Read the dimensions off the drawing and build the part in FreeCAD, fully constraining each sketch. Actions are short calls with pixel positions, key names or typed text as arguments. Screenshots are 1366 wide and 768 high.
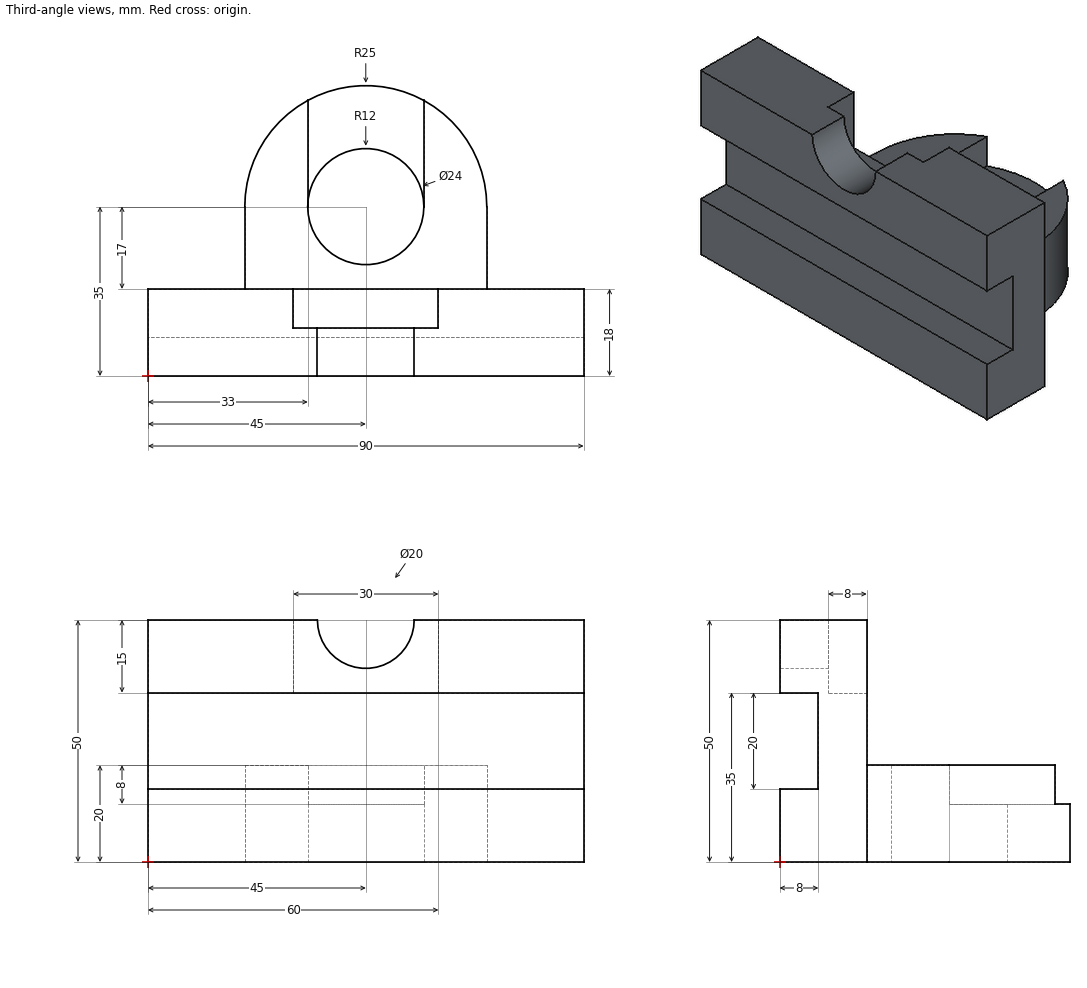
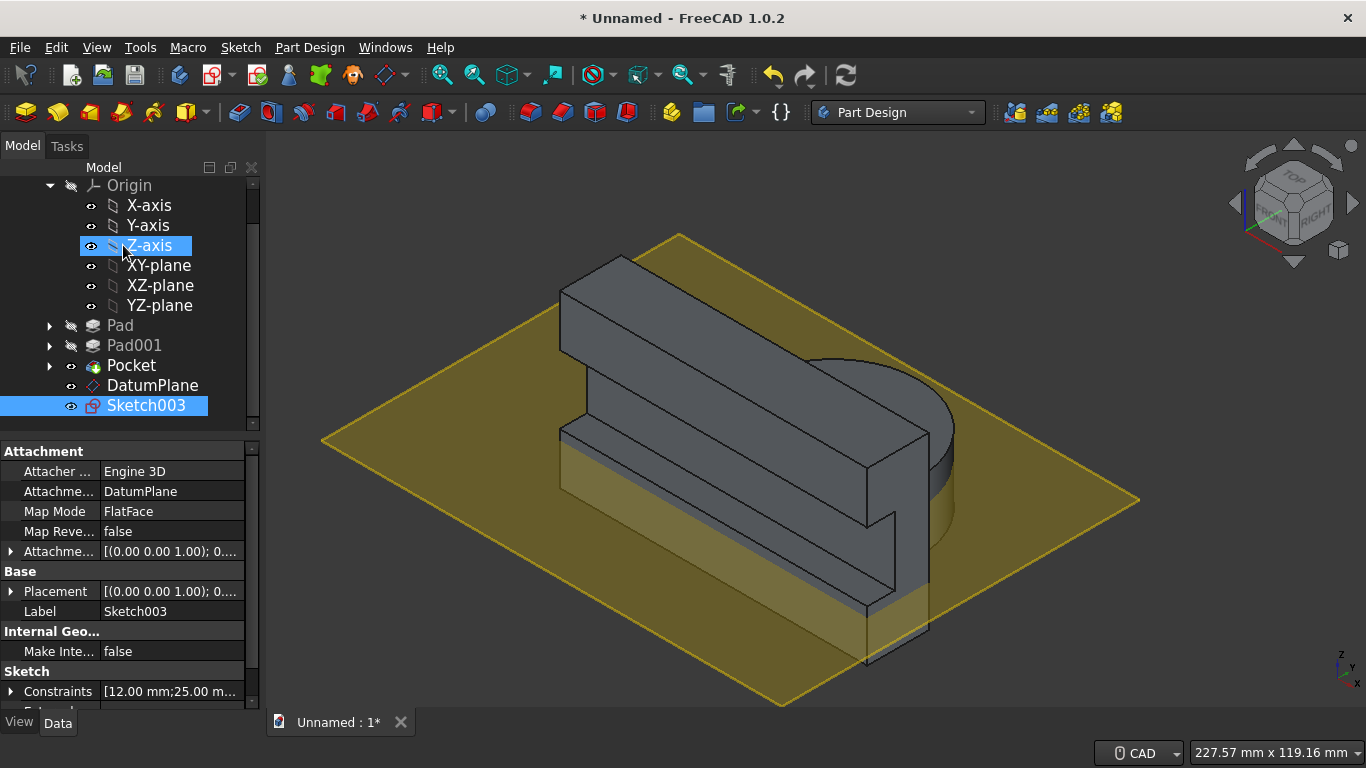
click(240, 112)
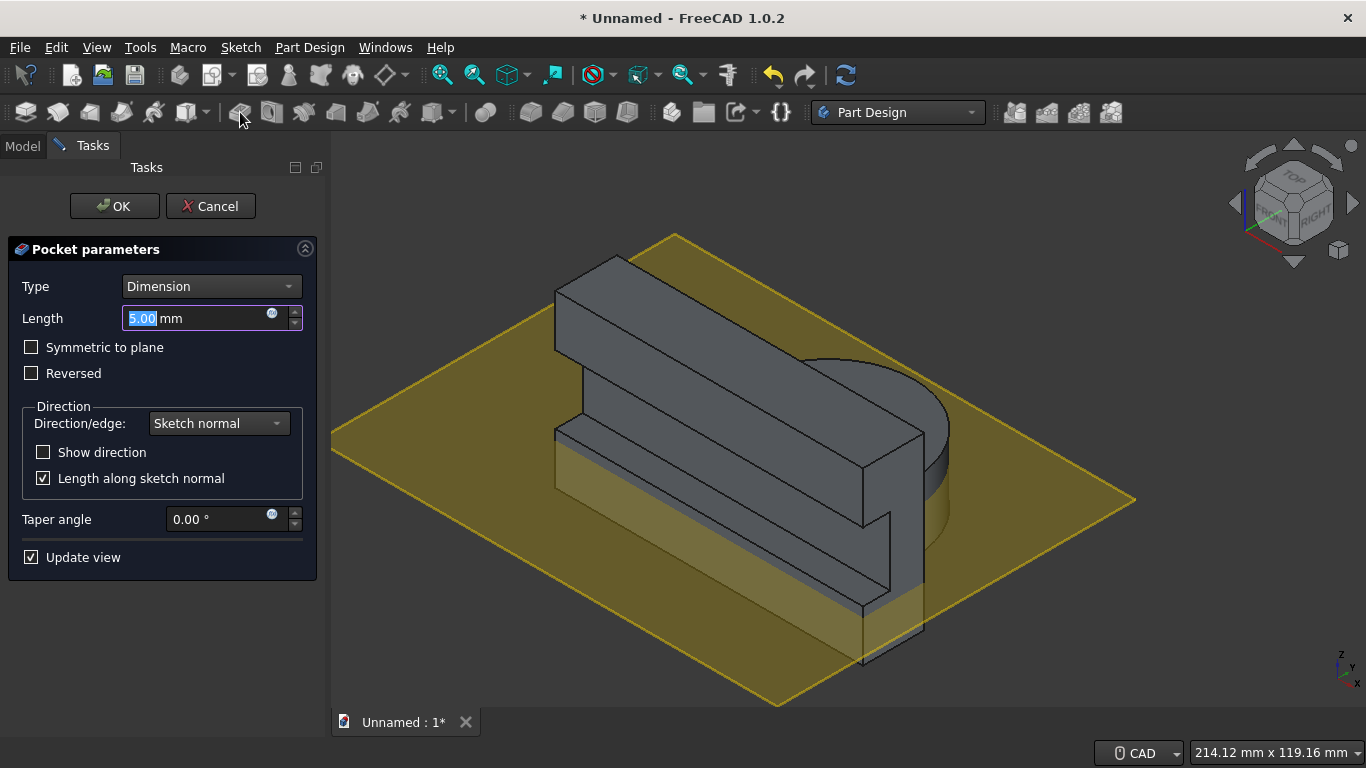
text(8)
key(Tab)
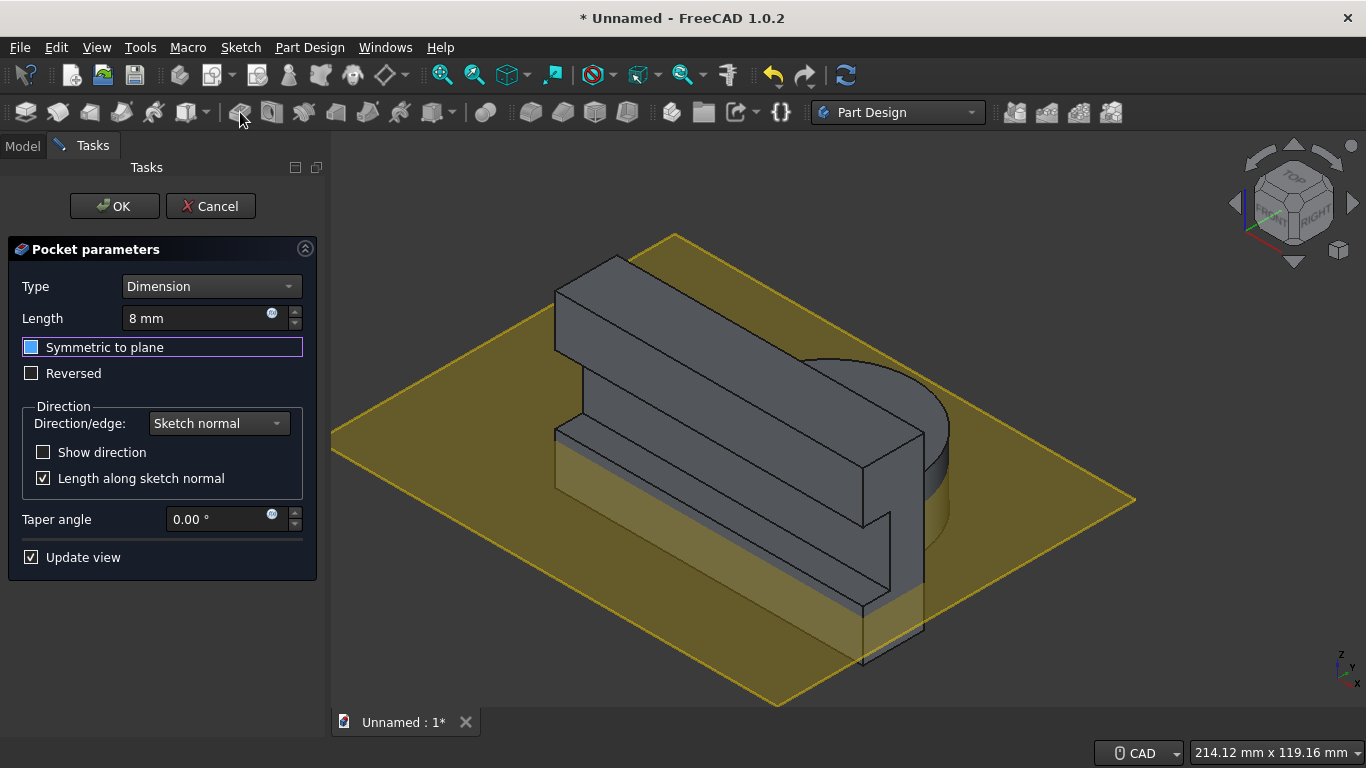
click(30, 373)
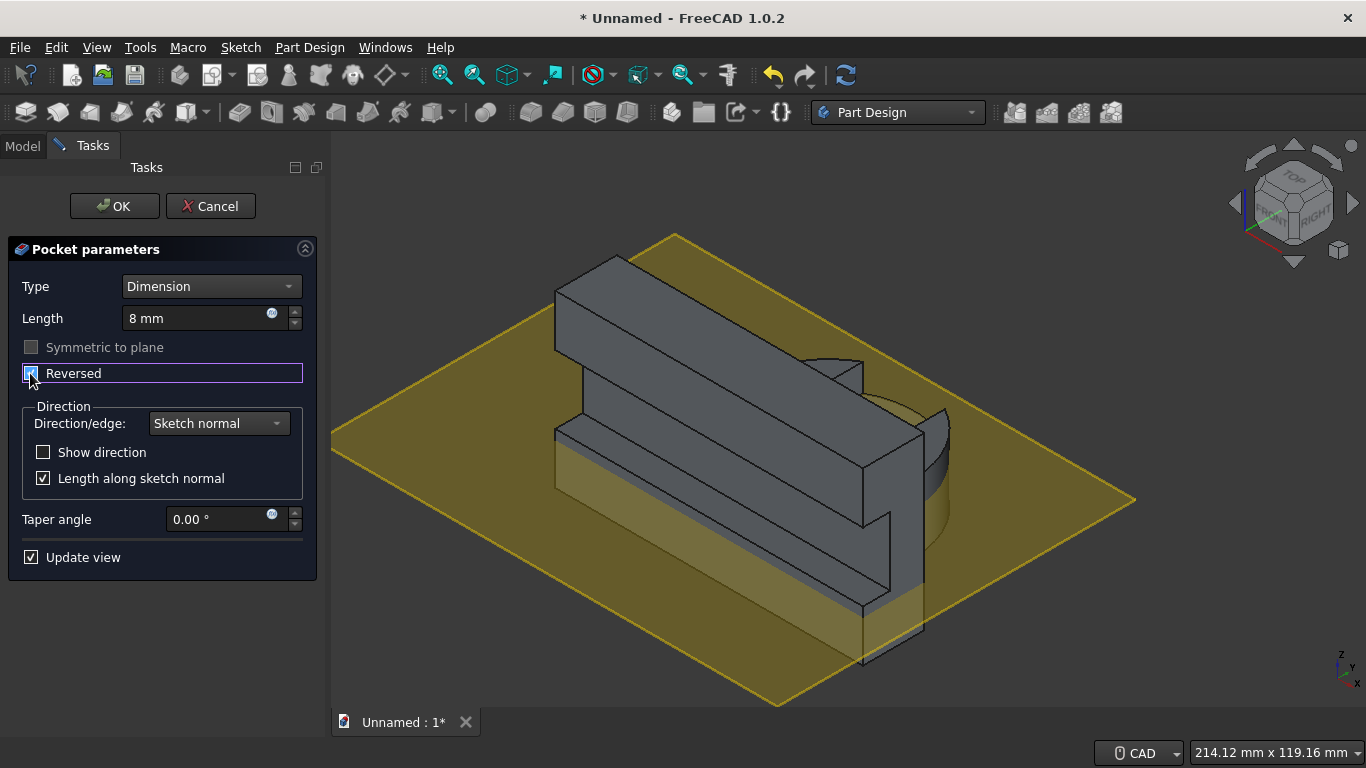
click(115, 206)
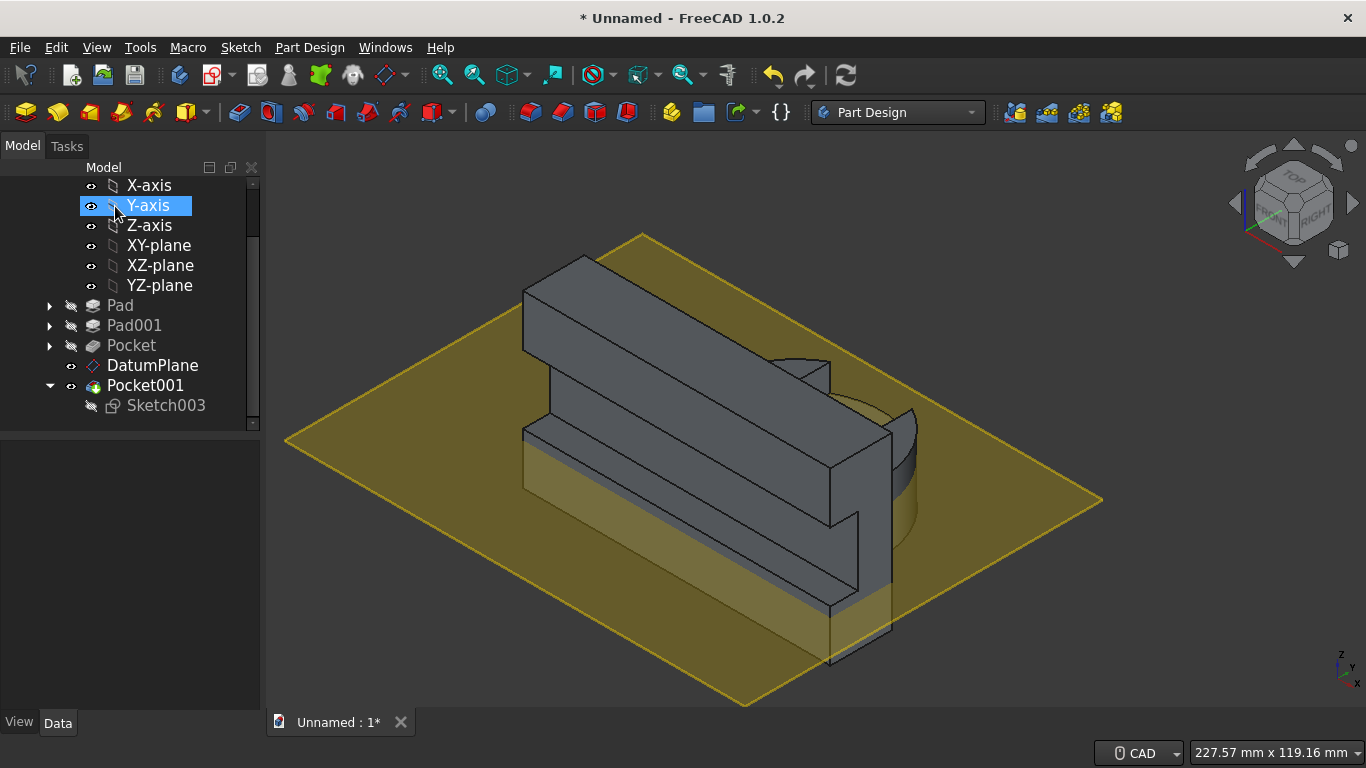
click(116, 366)
key(space)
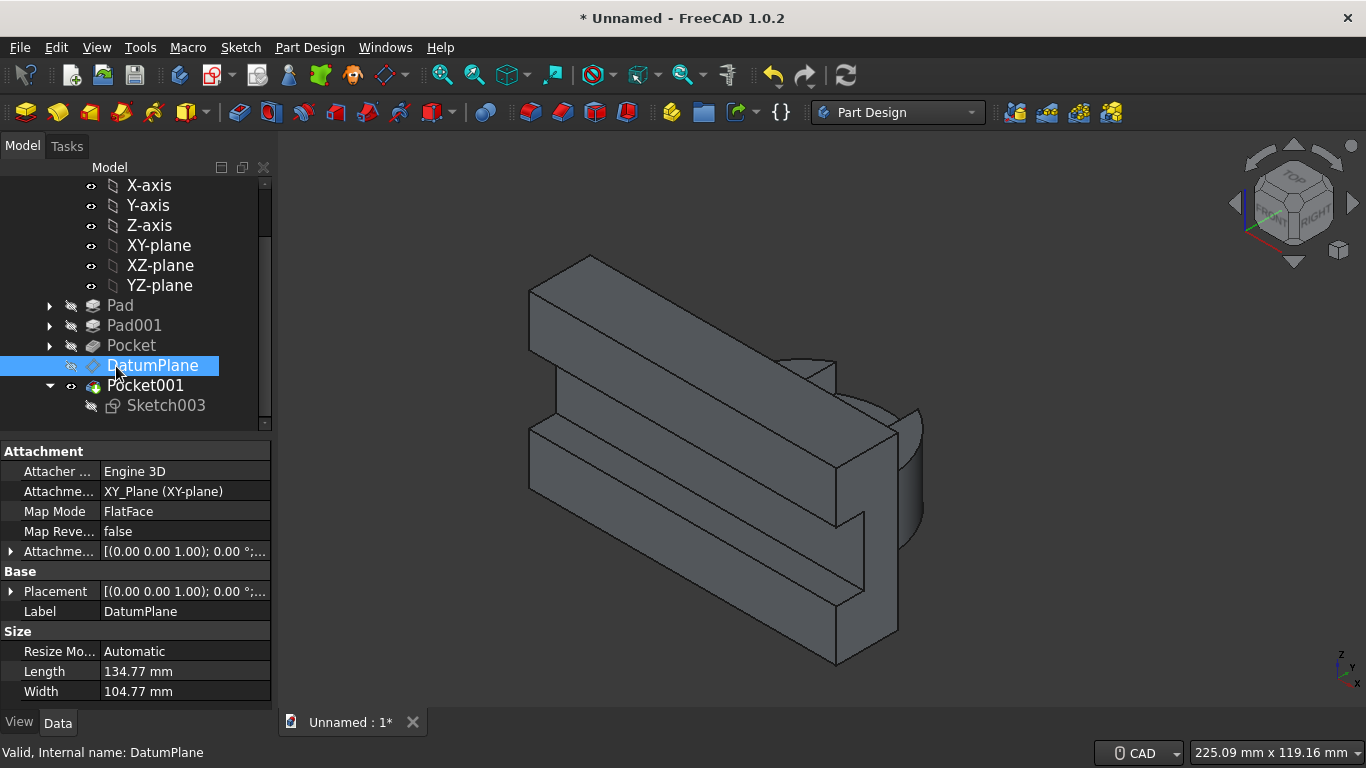
key(4)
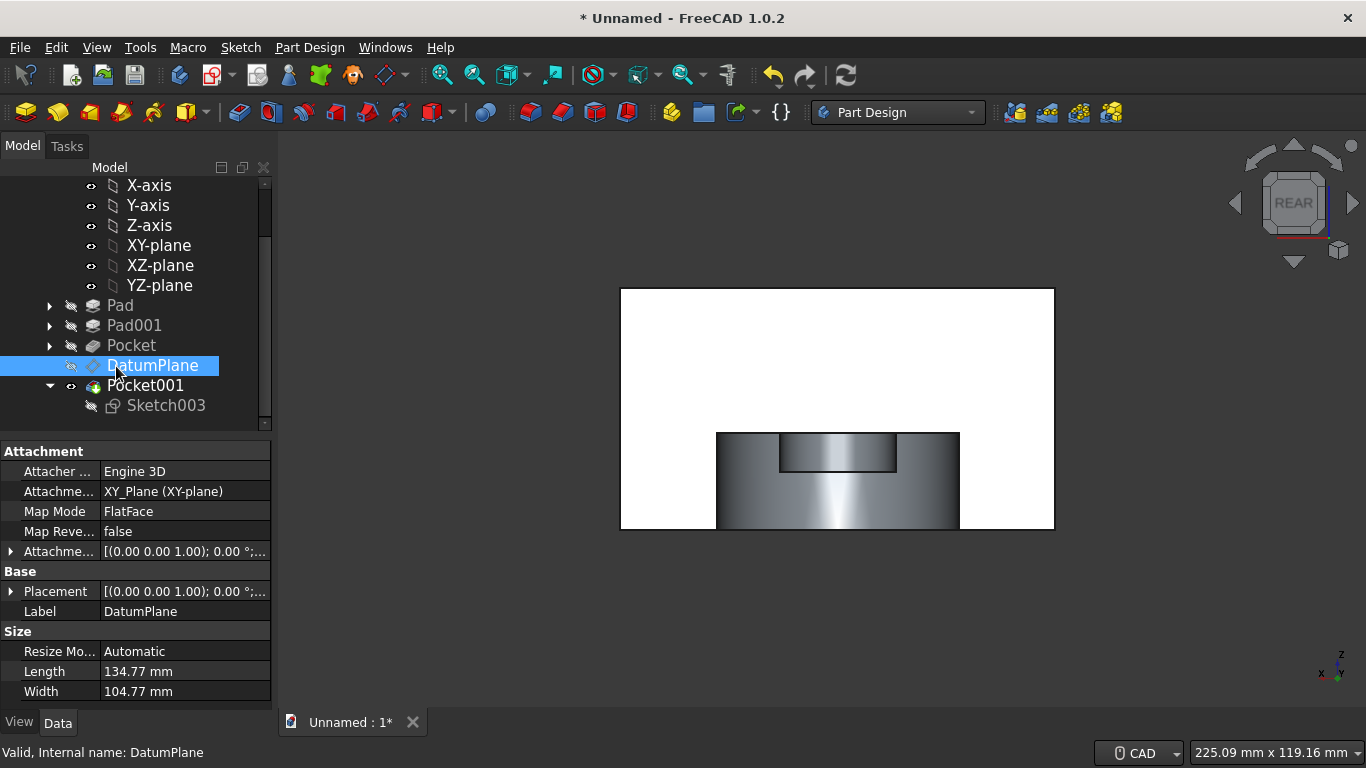
click(444, 76)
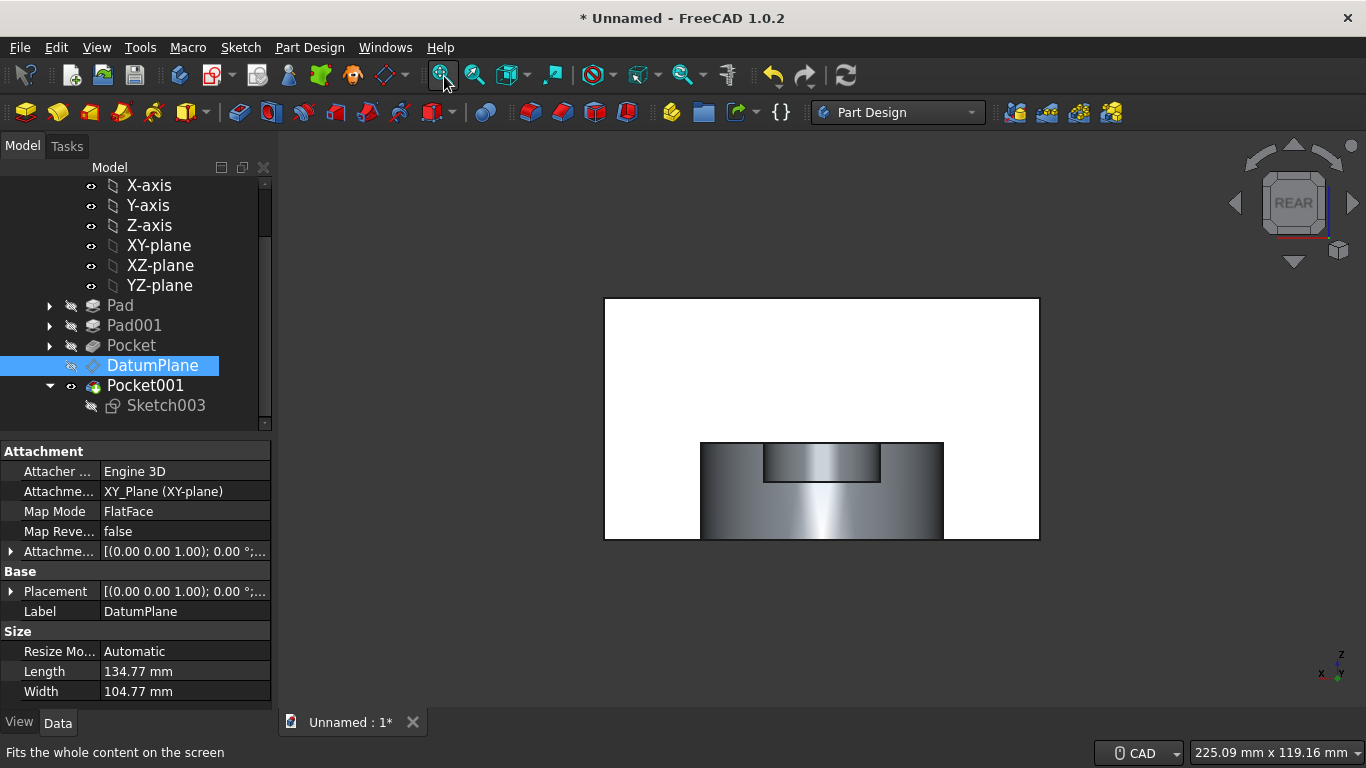
click(698, 383)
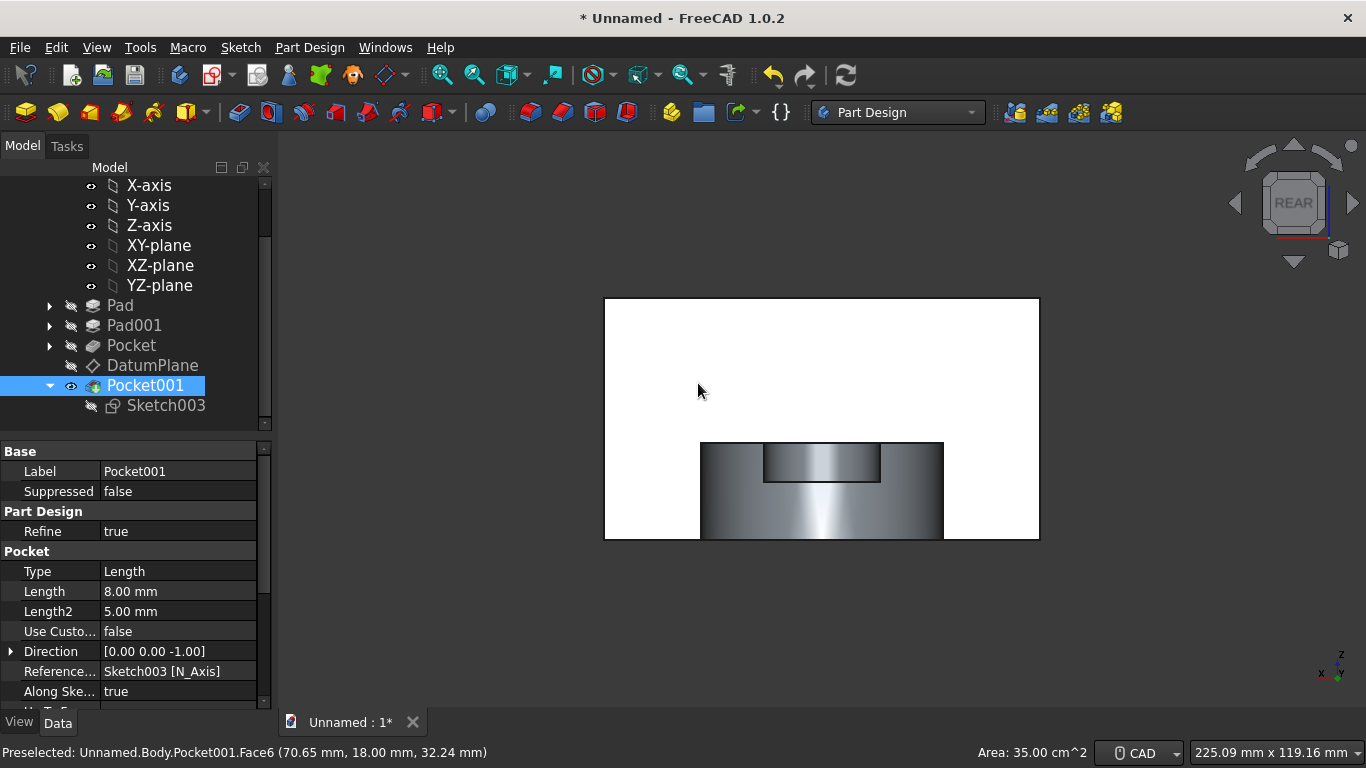
click(212, 76)